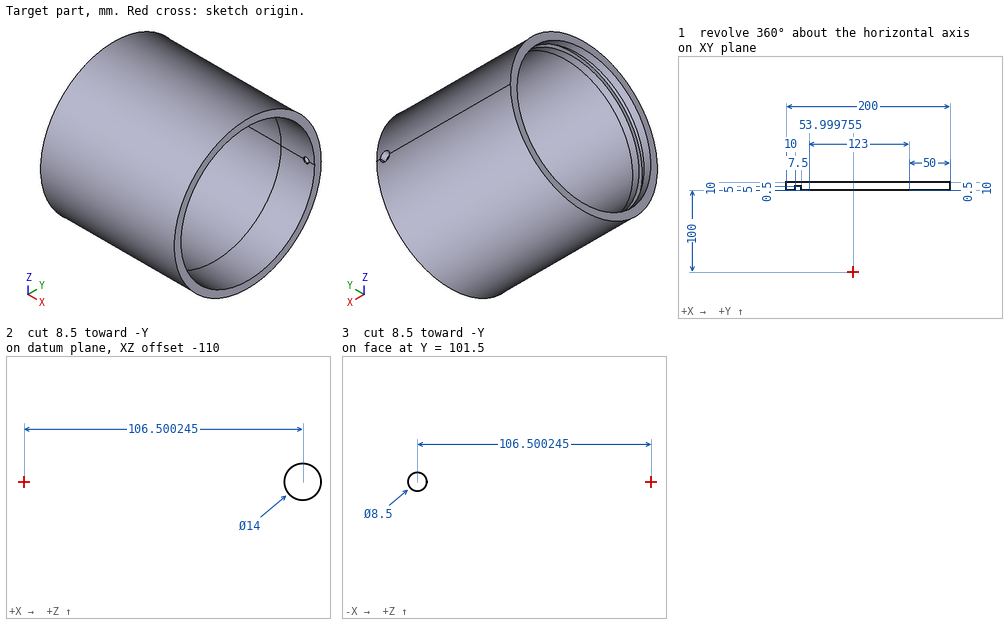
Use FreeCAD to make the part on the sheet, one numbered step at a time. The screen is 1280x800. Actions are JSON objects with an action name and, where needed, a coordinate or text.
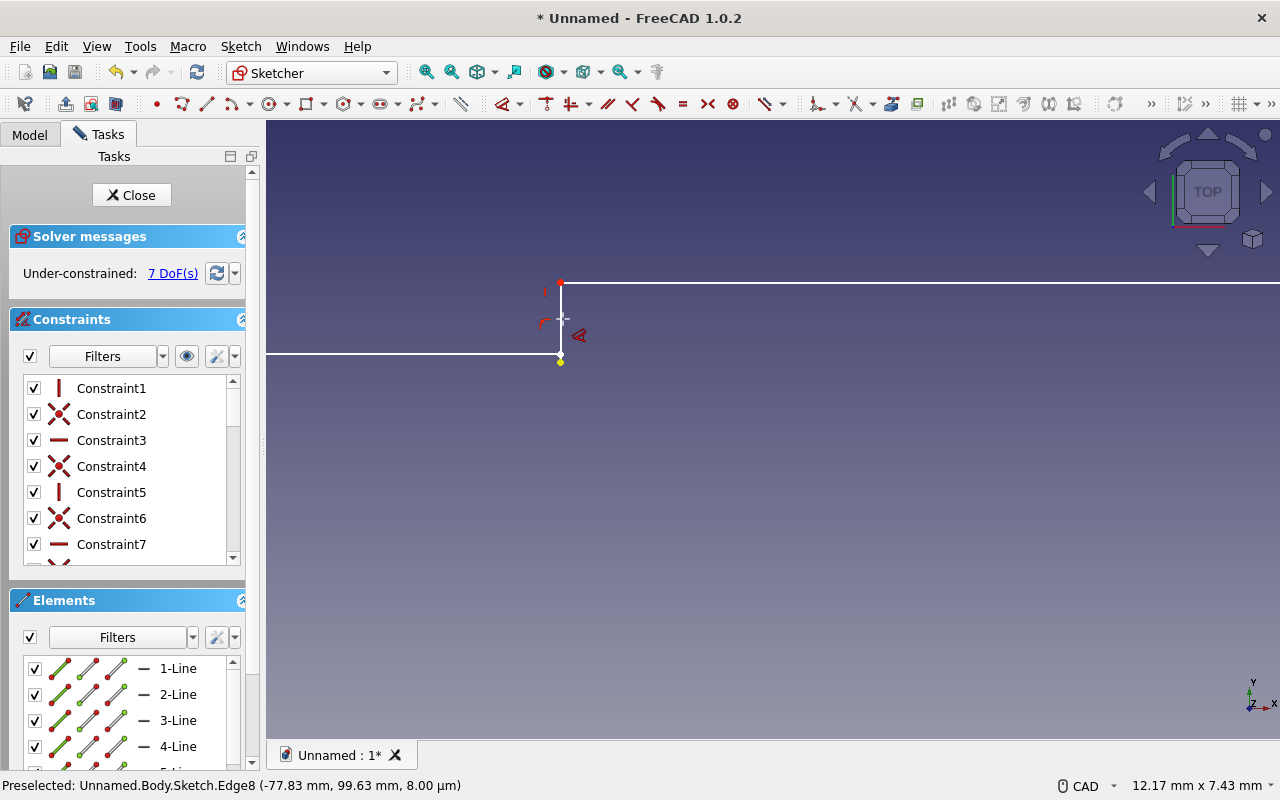
{"action": "left_click", "coordinate": [561, 315]}
{"action": "left_click", "coordinate": [527, 323]}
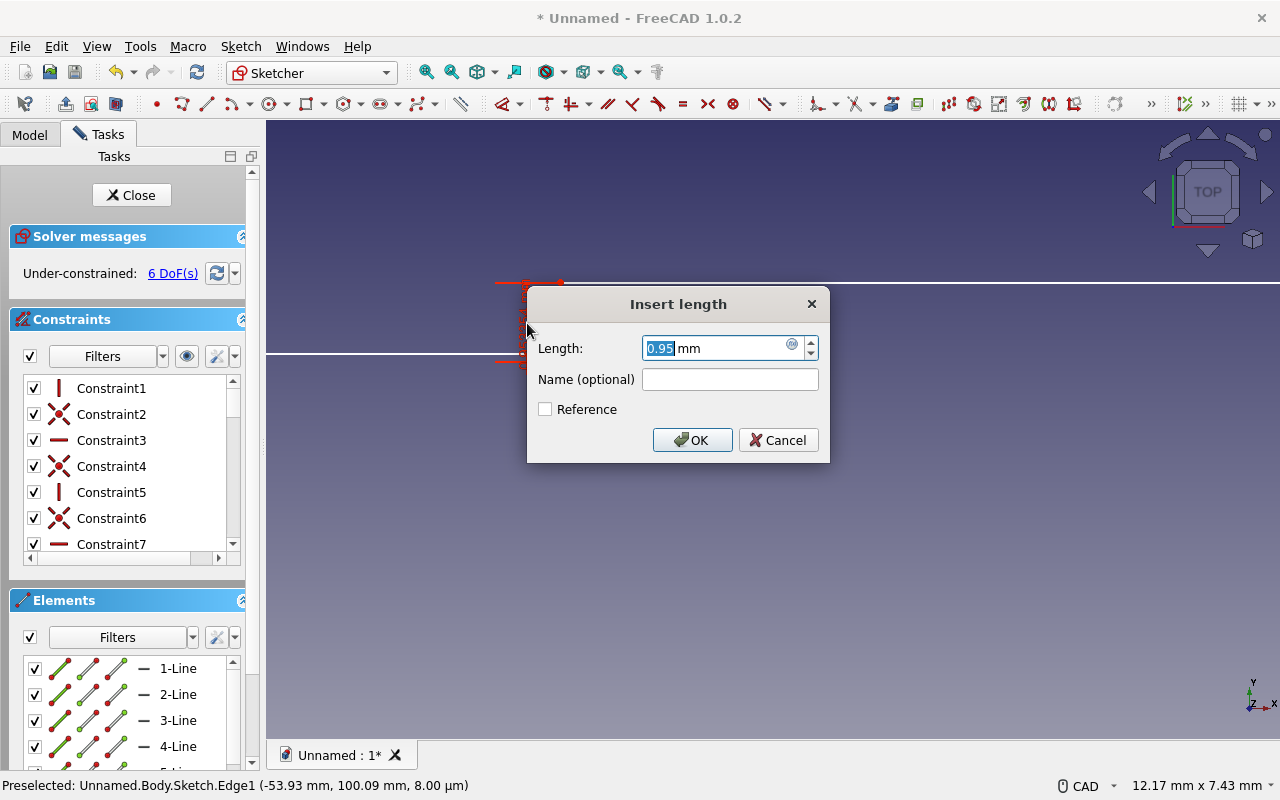
{"action": "type", "text": "0.5"}
{"action": "key", "text": "Return"}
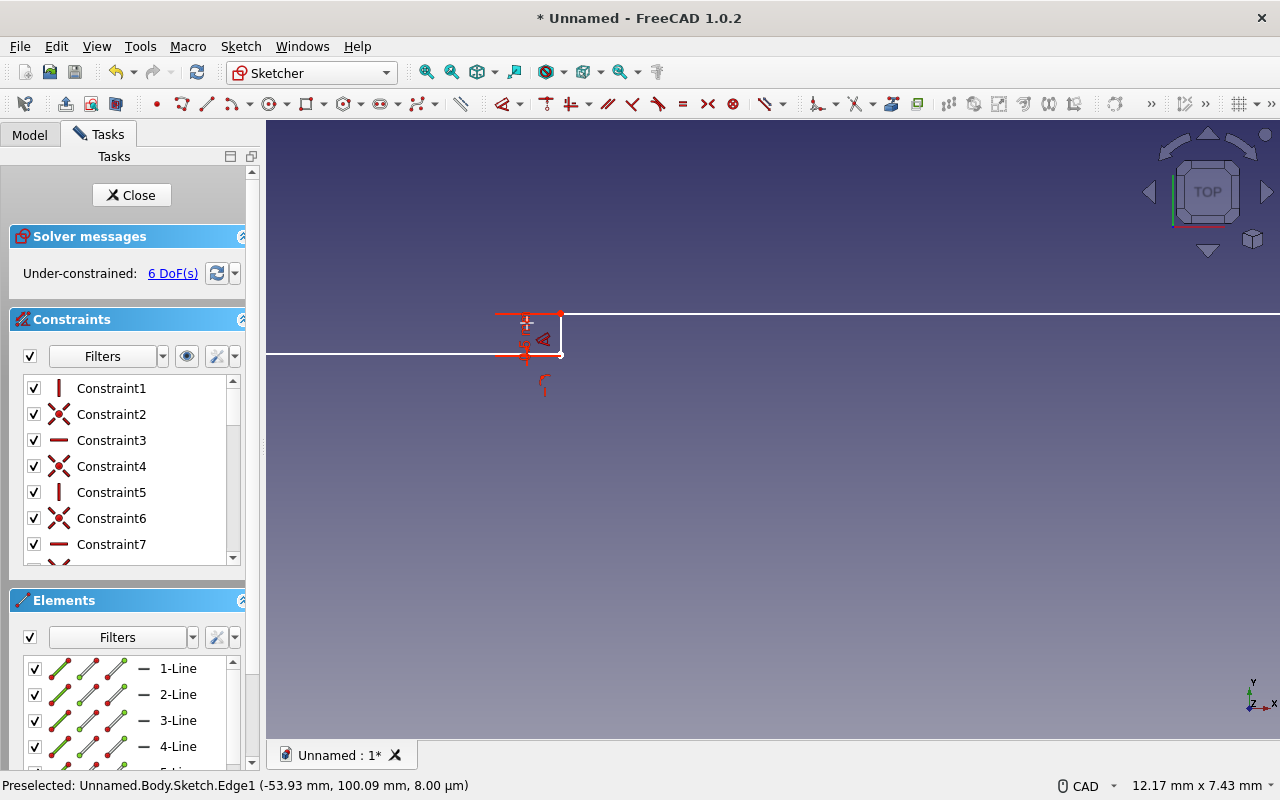
{"action": "scroll", "coordinate": [452, 275], "scroll_direction": "down", "scroll_amount": 16}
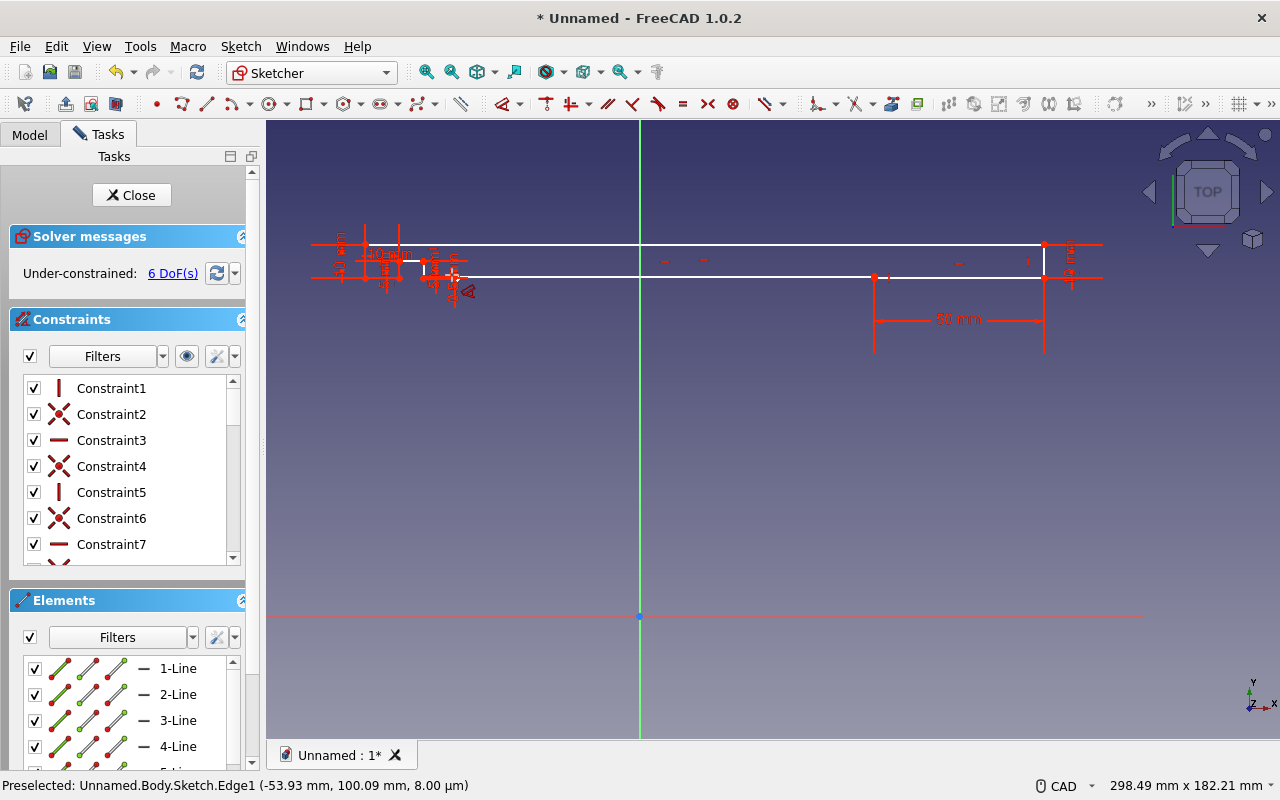
{"action": "left_click", "coordinate": [582, 277]}
{"action": "left_click", "coordinate": [665, 311]}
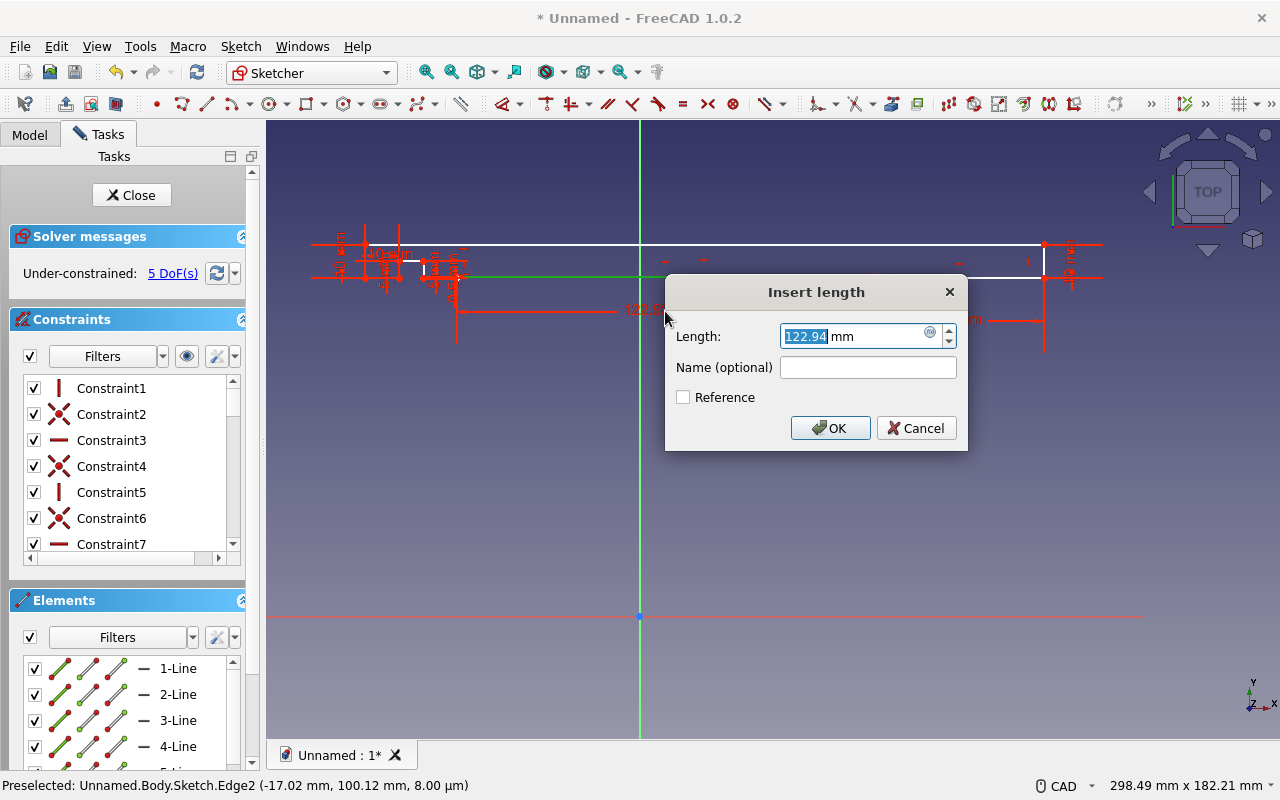
{"action": "type", "text": "123"}
{"action": "key", "text": "Return"}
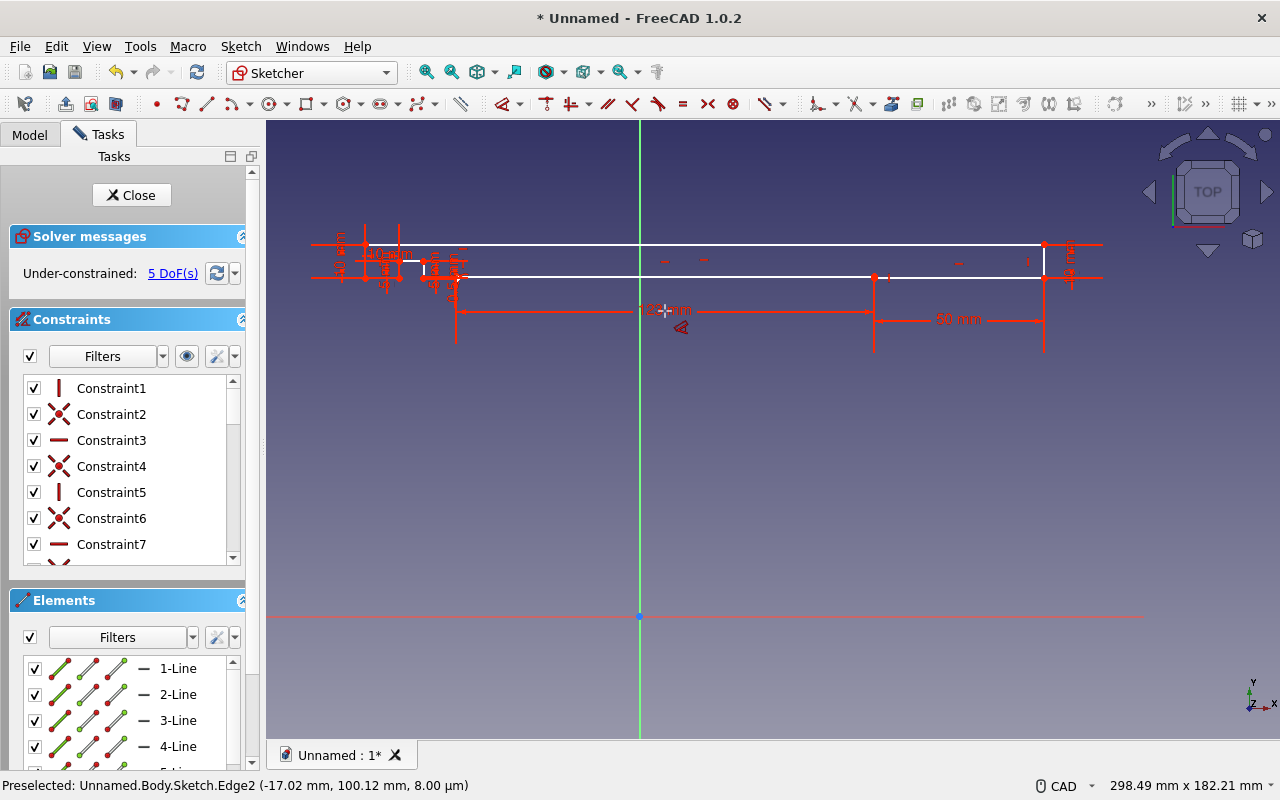
{"action": "scroll", "coordinate": [874, 278], "scroll_direction": "up", "scroll_amount": 16}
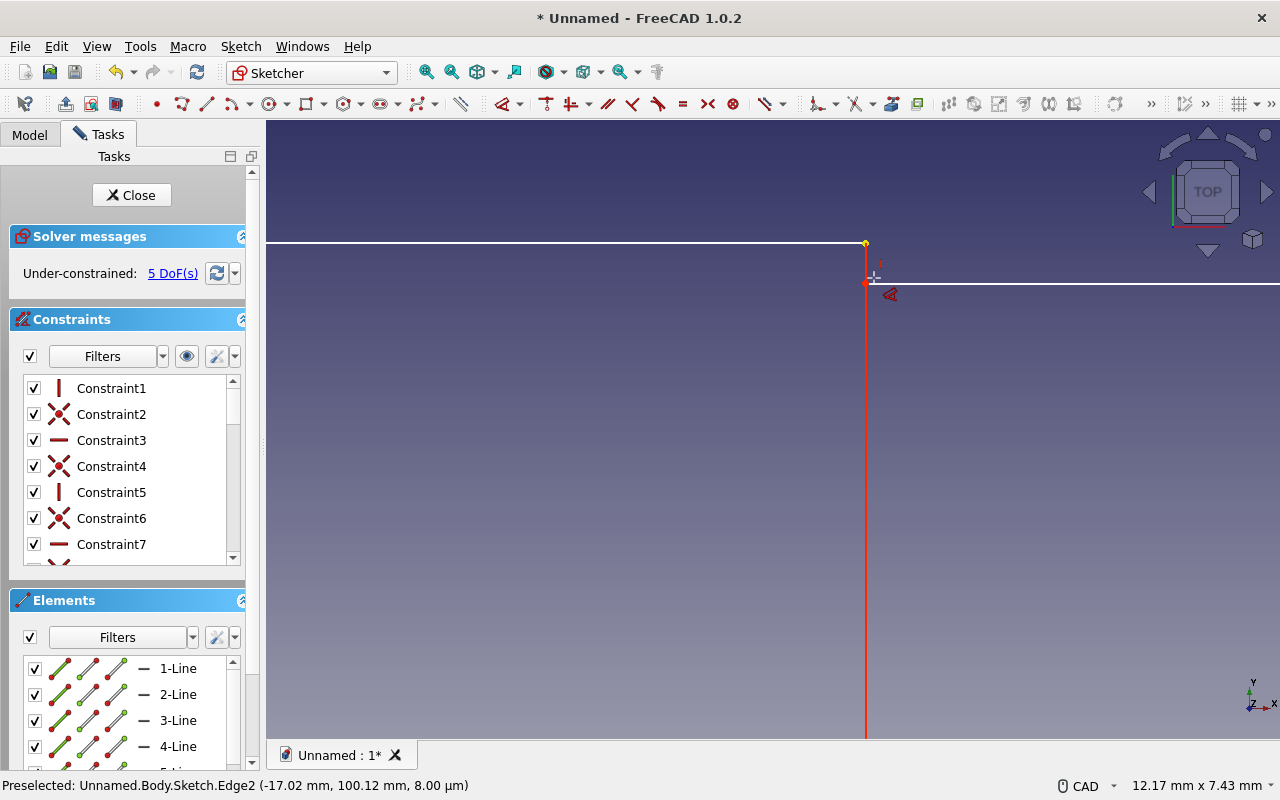
{"action": "left_click", "coordinate": [866, 263]}
{"action": "left_click", "coordinate": [900, 263]}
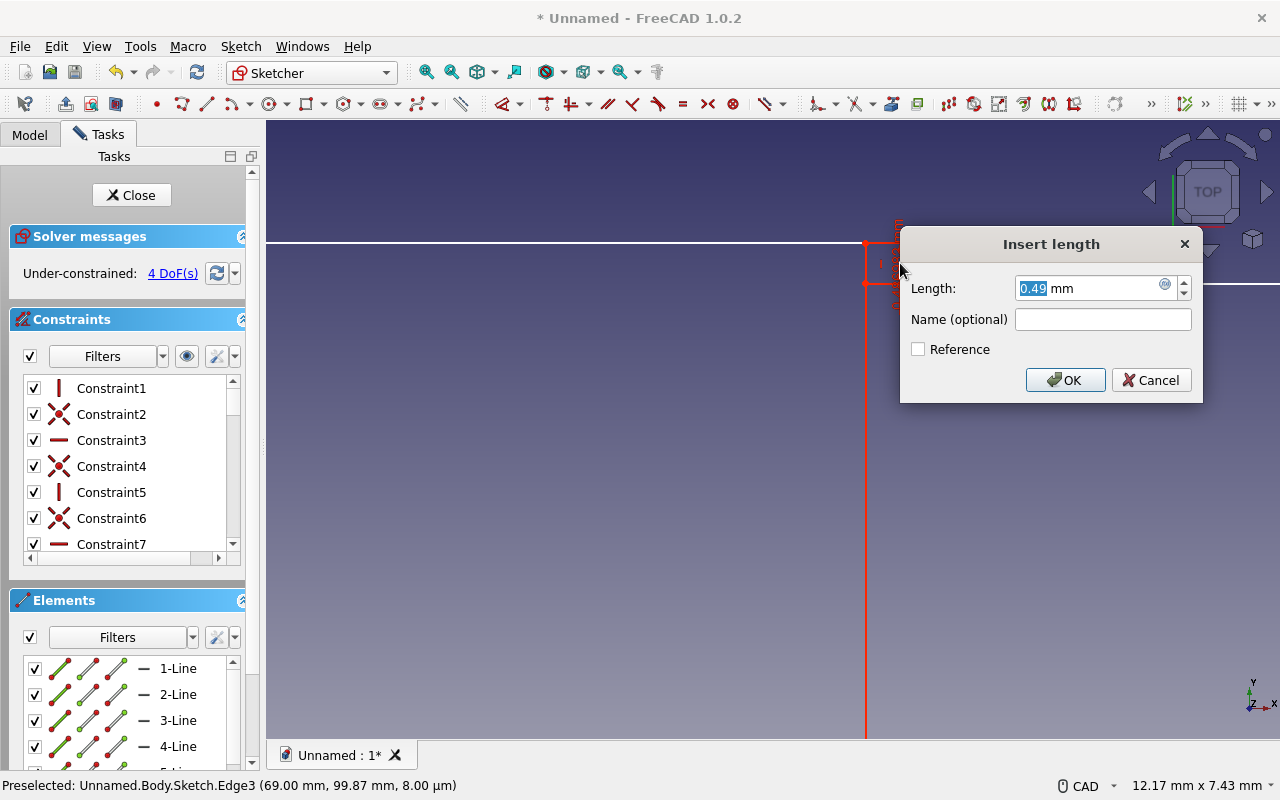
{"action": "type", "text": "0.5"}
{"action": "key", "text": "Return"}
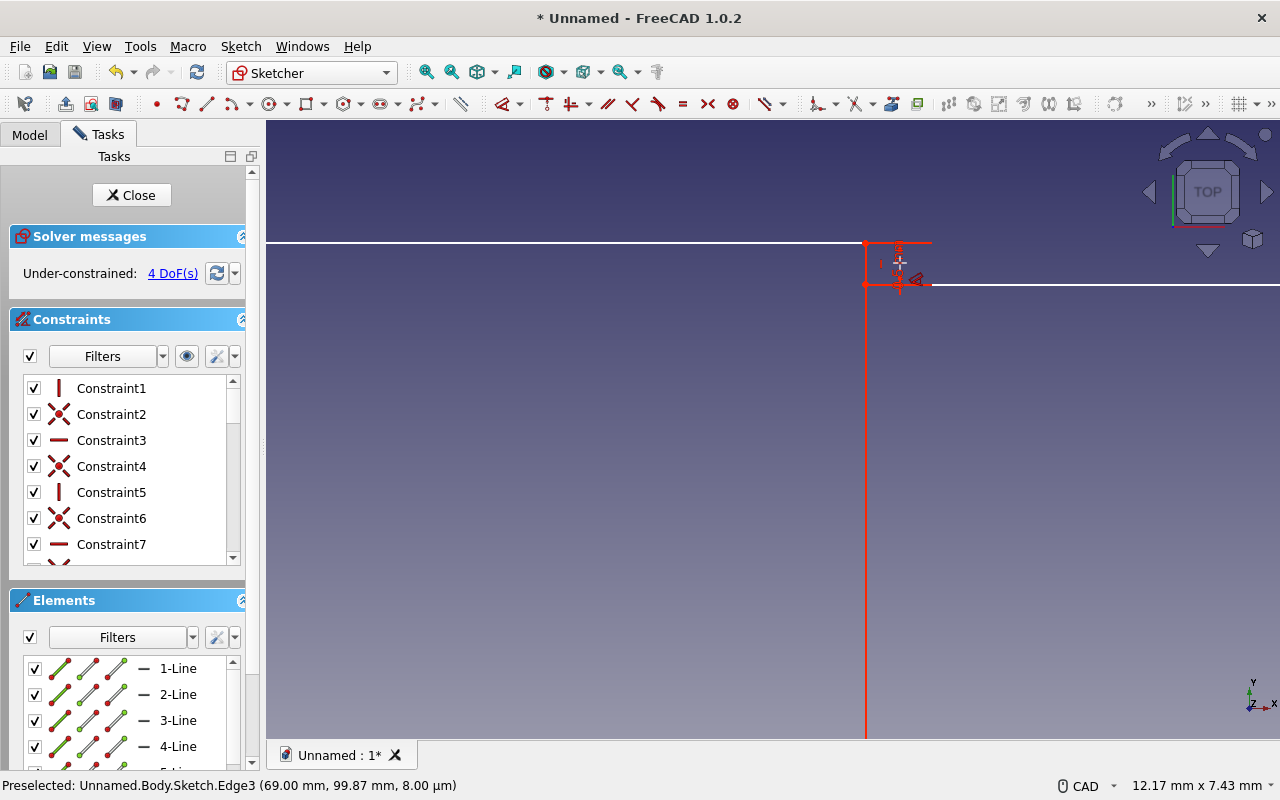
{"action": "scroll", "coordinate": [875, 278], "scroll_direction": "down", "scroll_amount": 16}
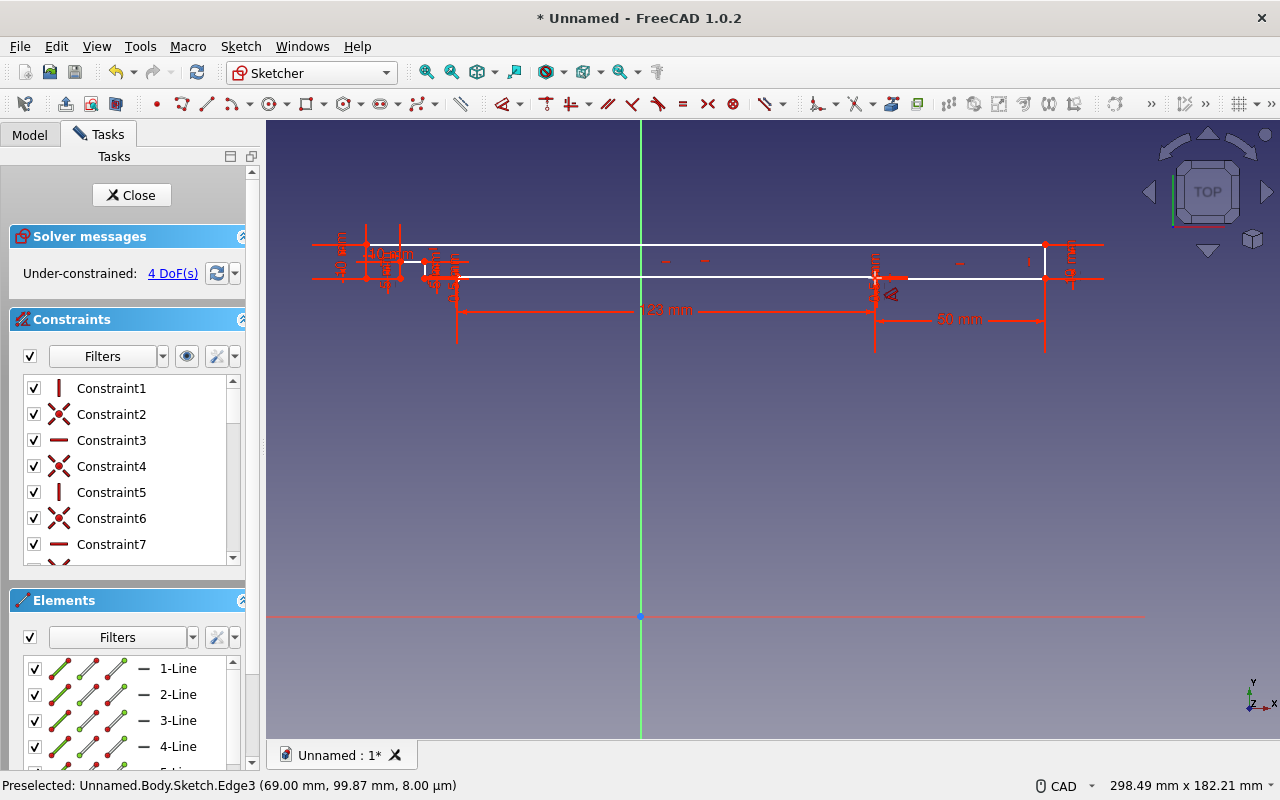
{"action": "left_click", "coordinate": [841, 245]}
{"action": "left_click", "coordinate": [706, 211]}